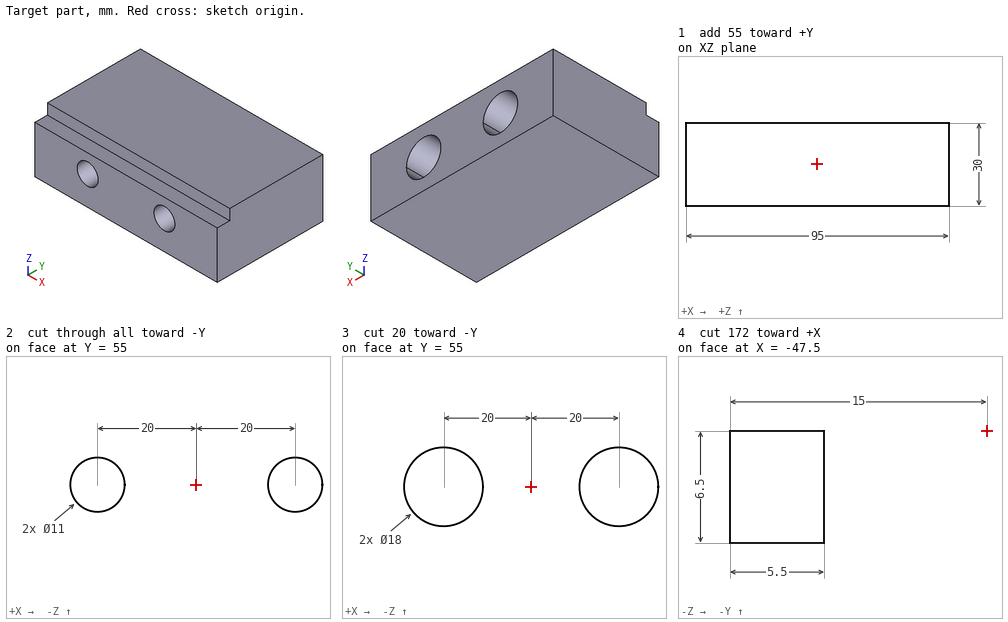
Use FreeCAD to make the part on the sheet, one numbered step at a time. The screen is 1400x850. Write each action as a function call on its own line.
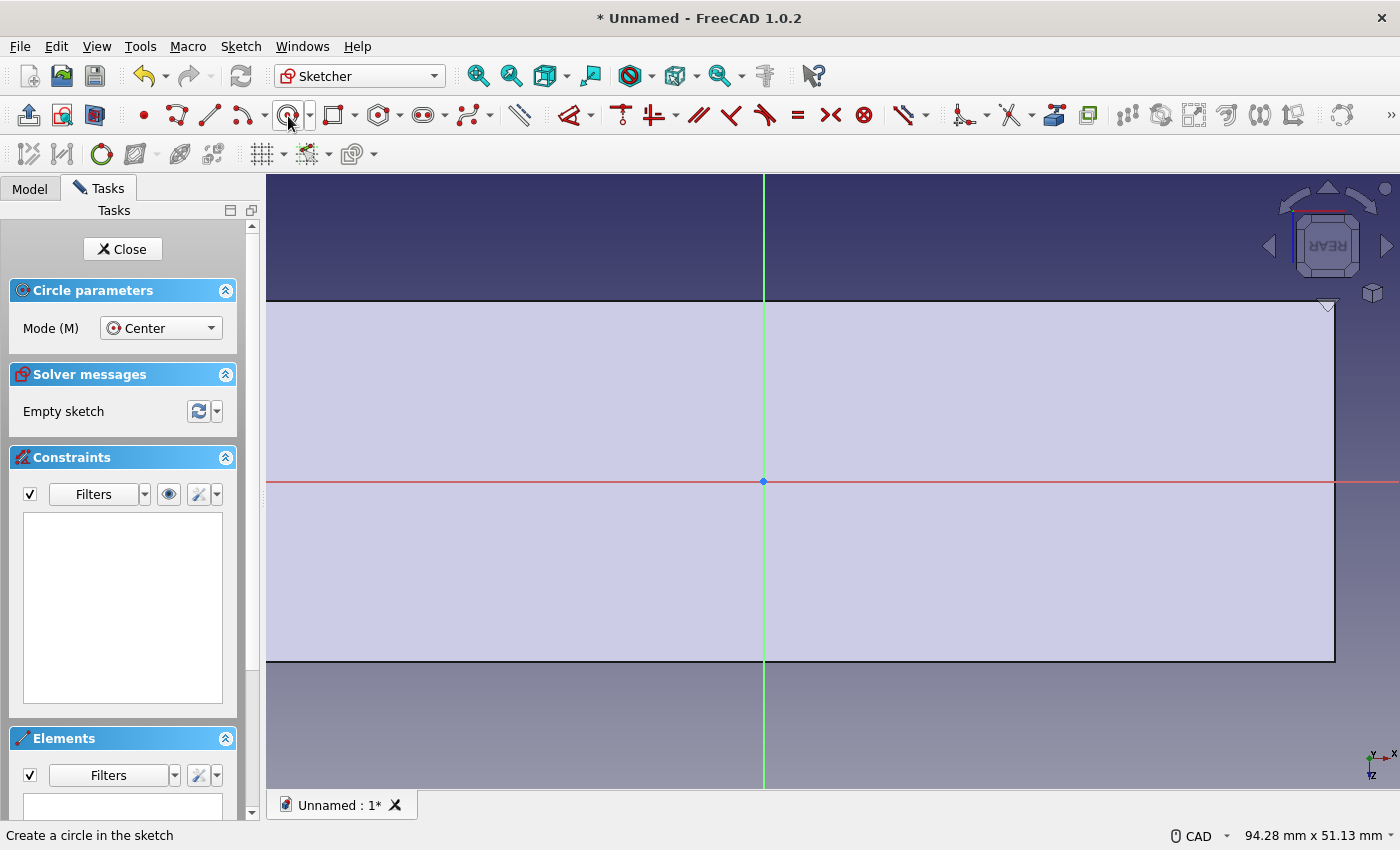
click(523, 481)
move(570, 435)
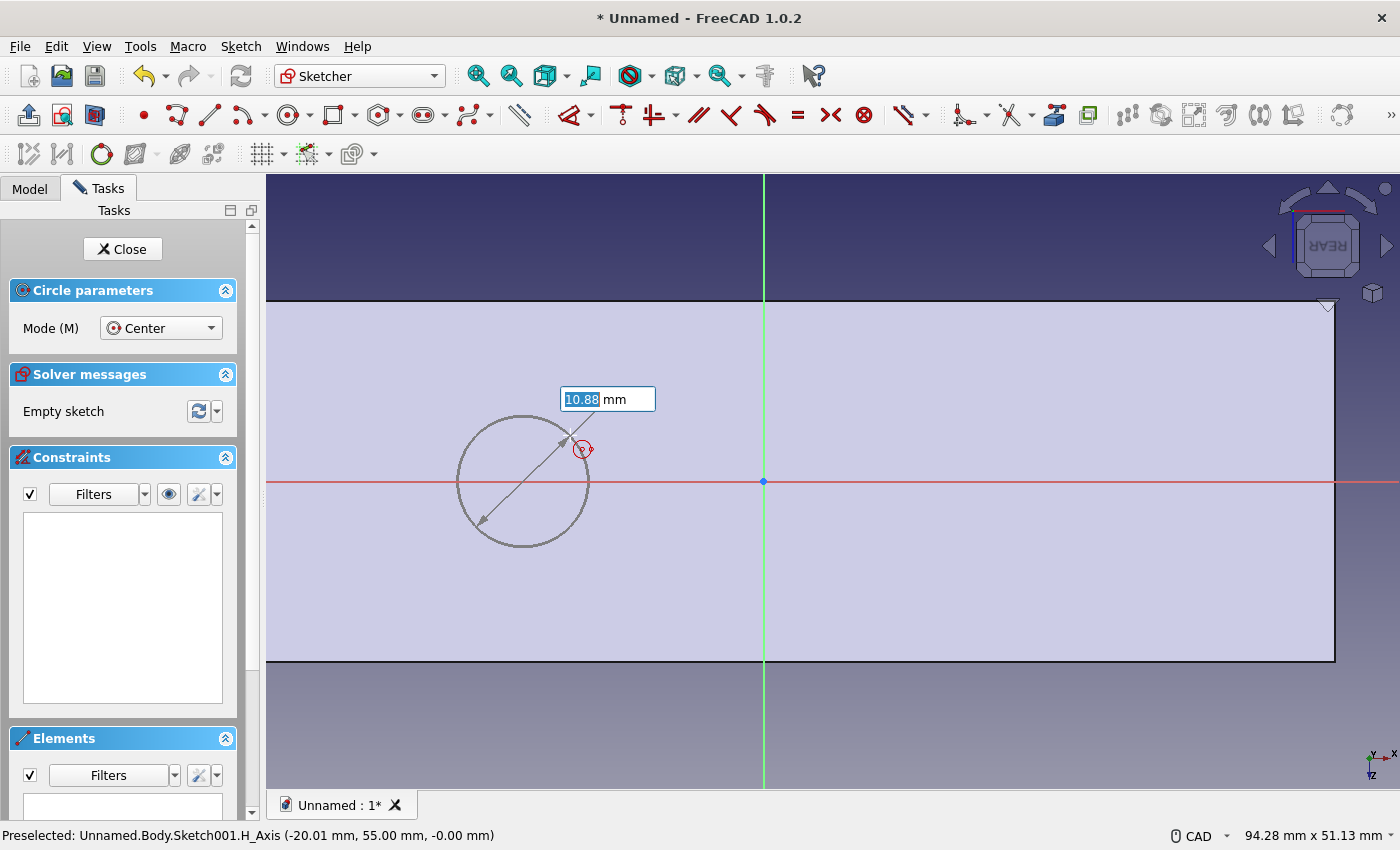
text(11)
key(Return)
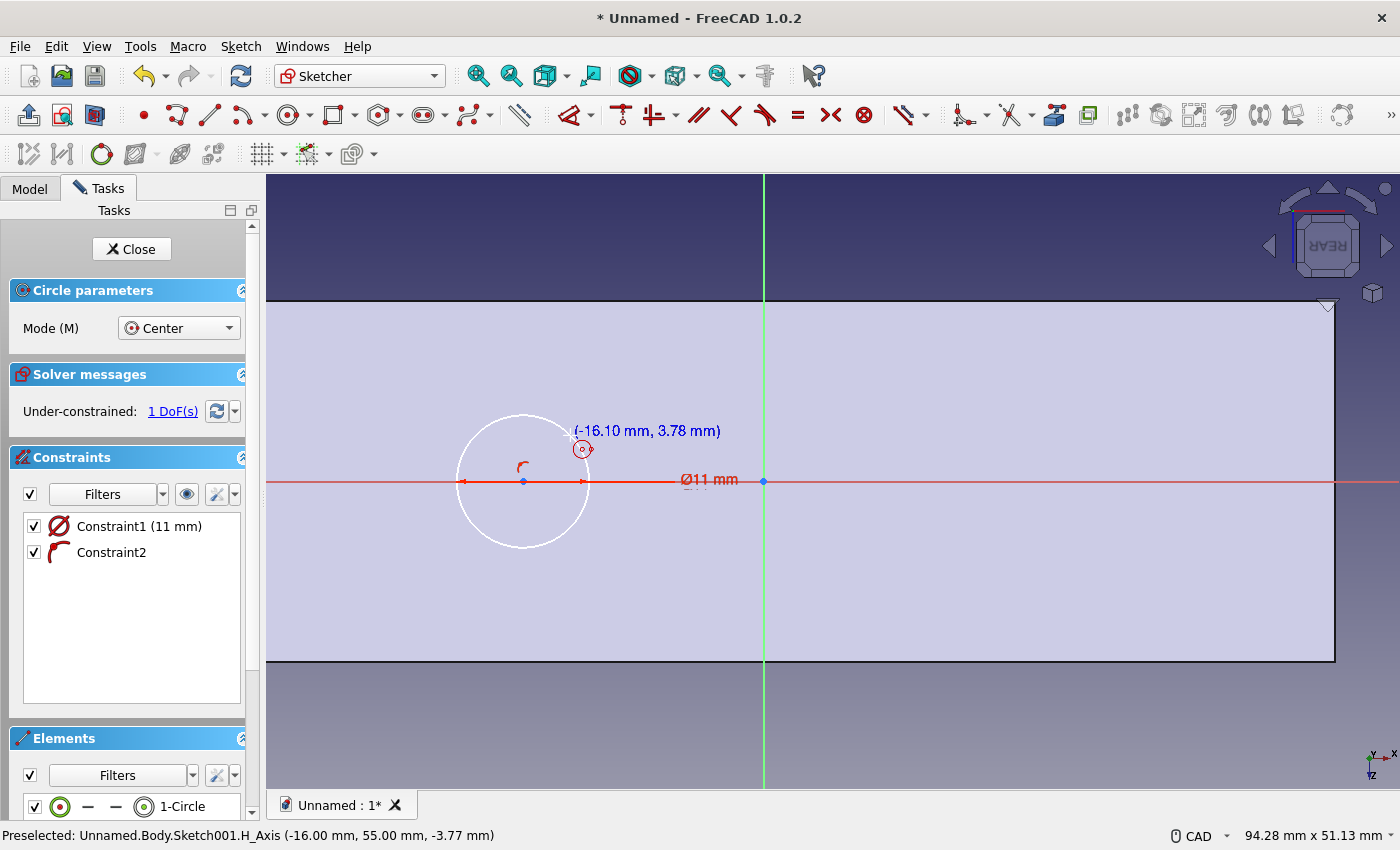
click(1004, 481)
move(1051, 435)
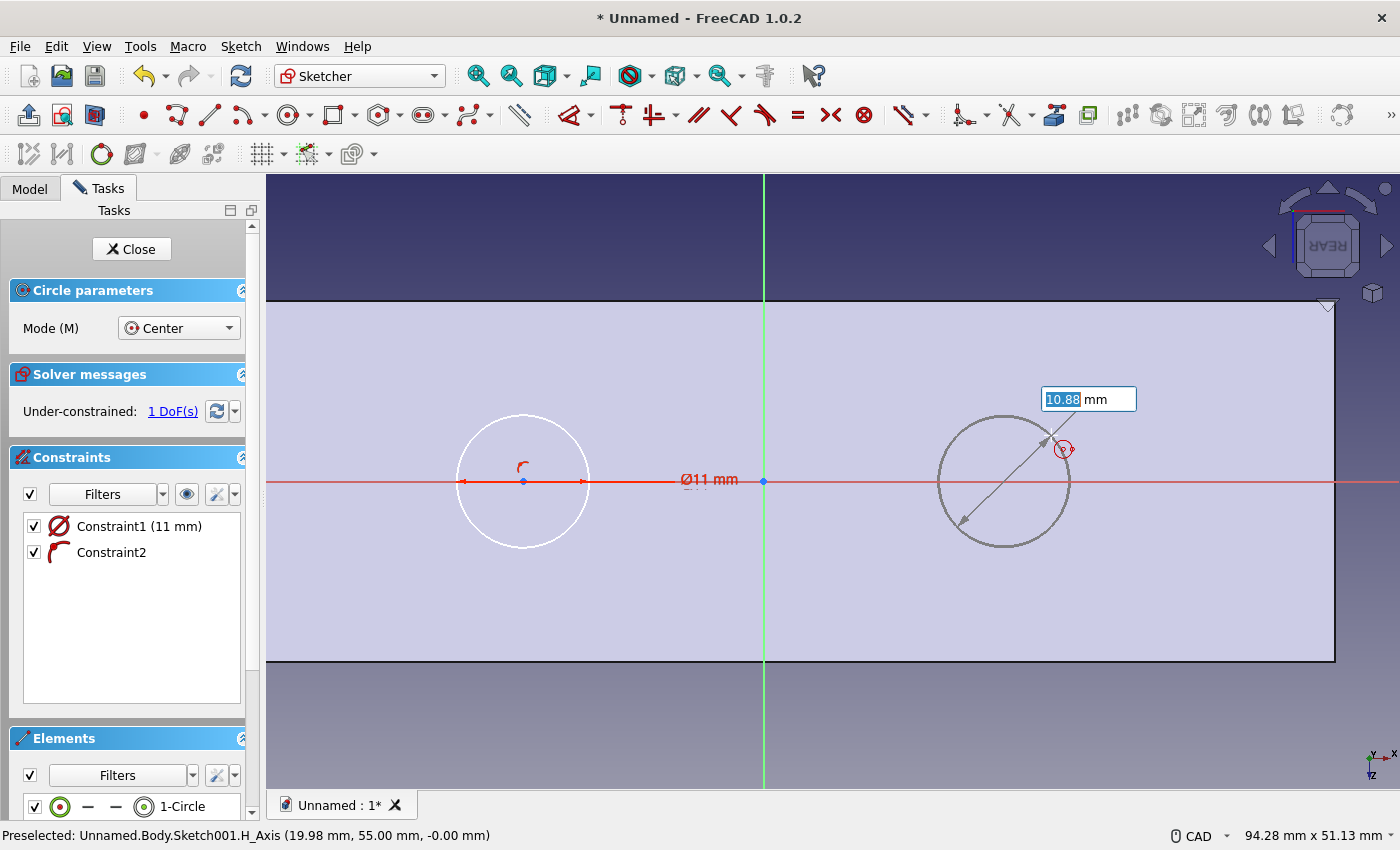
text(11)
key(Return)
key(Escape)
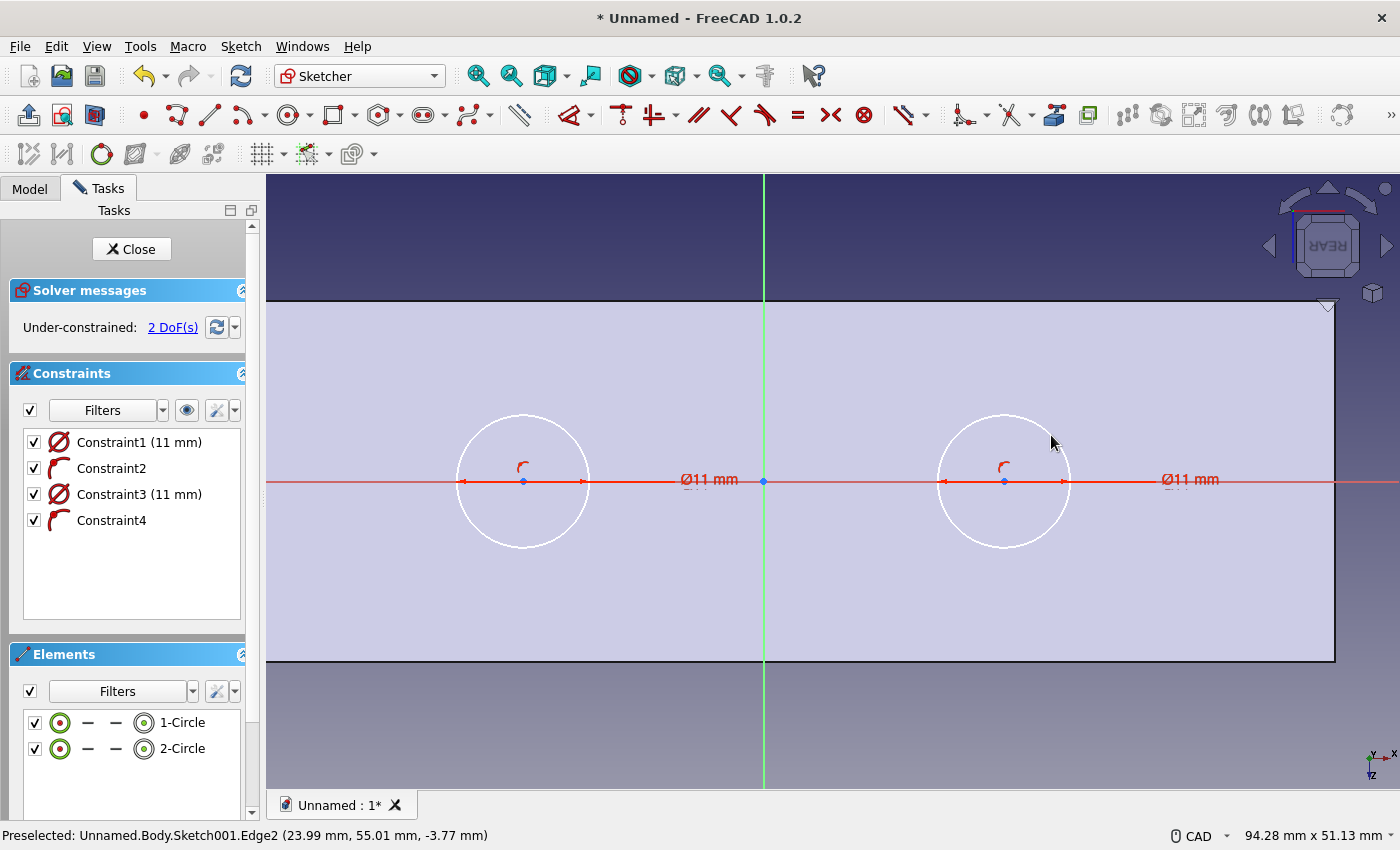
click(568, 116)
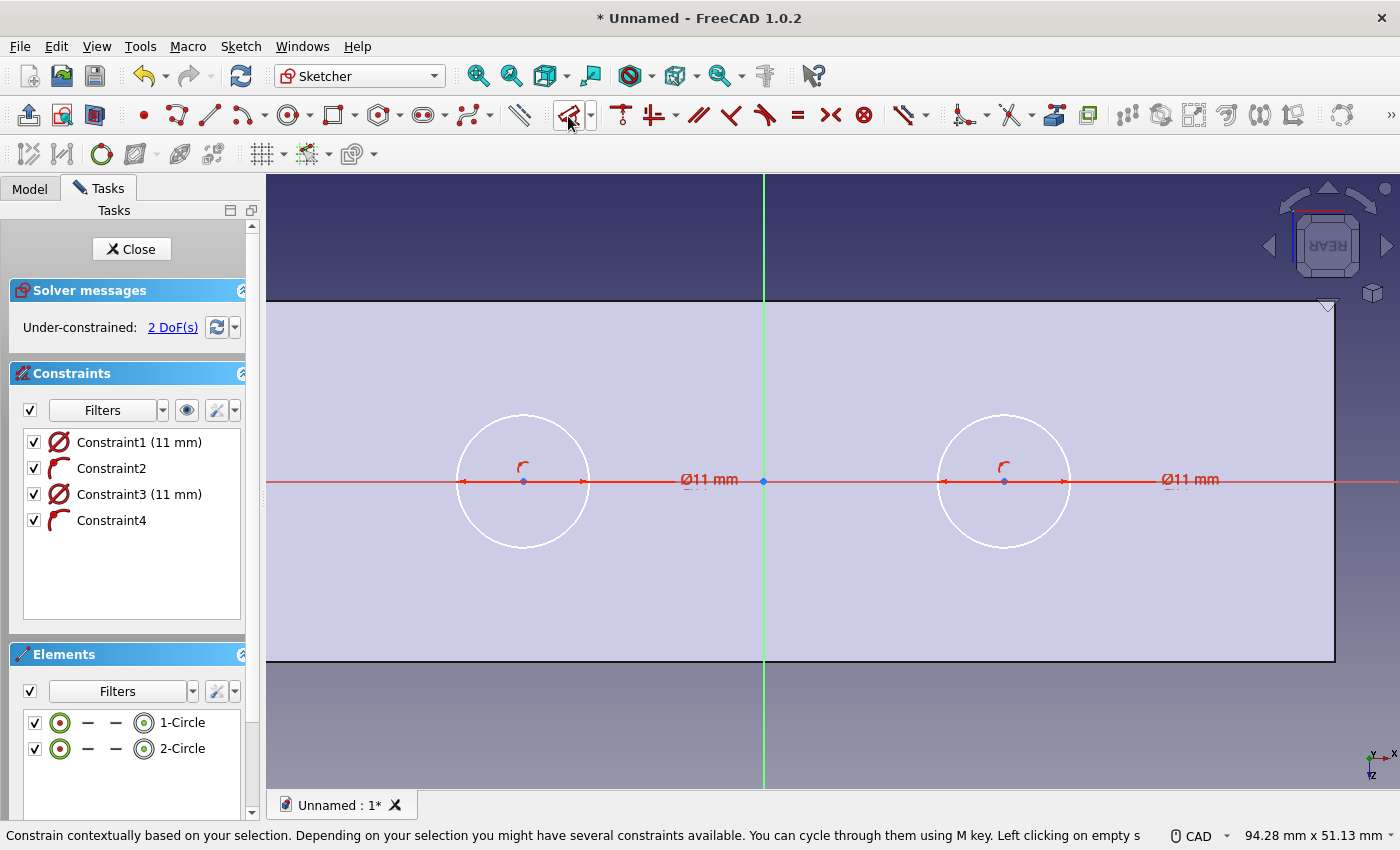
click(523, 481)
click(643, 515)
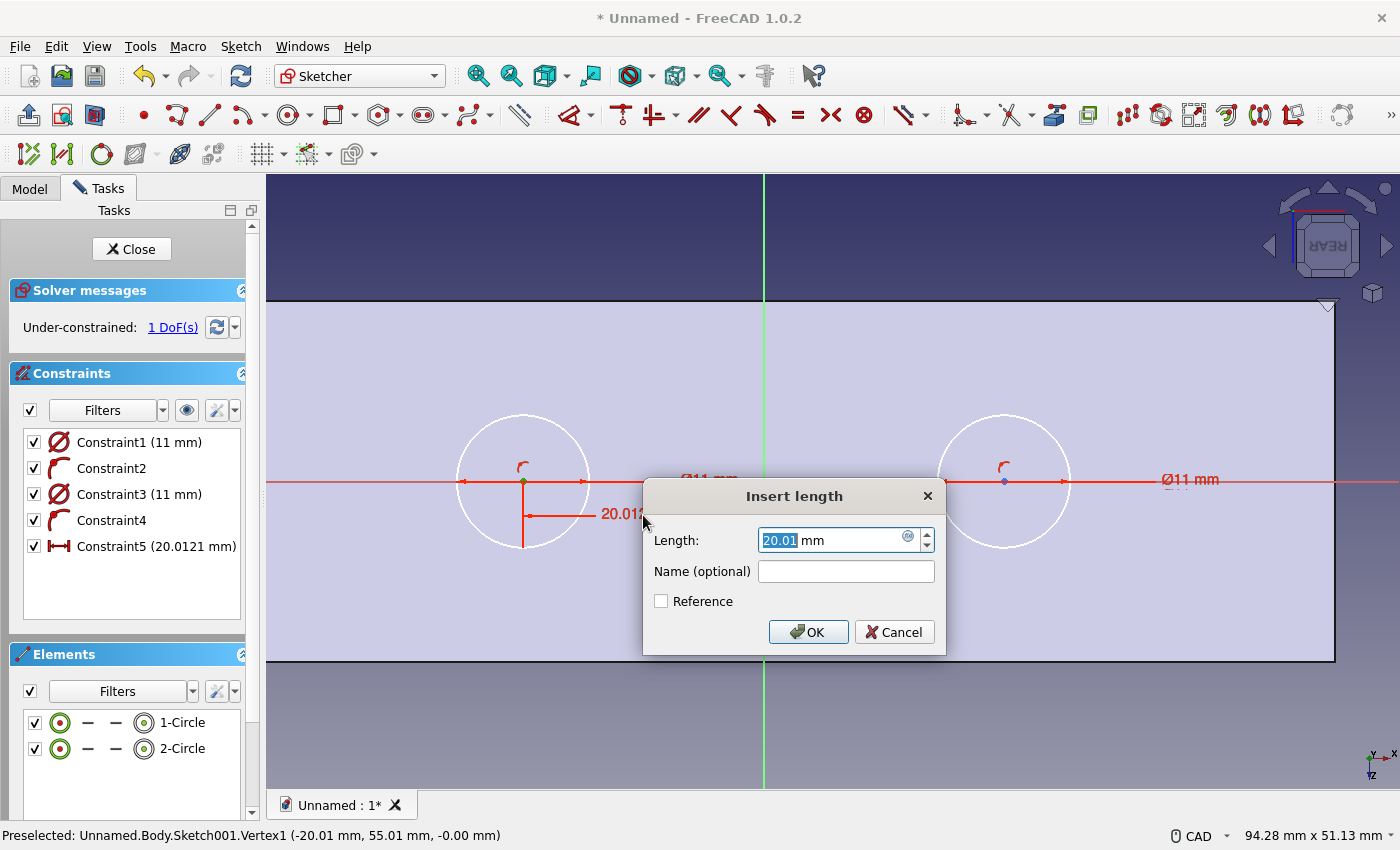
text(20)
key(Return)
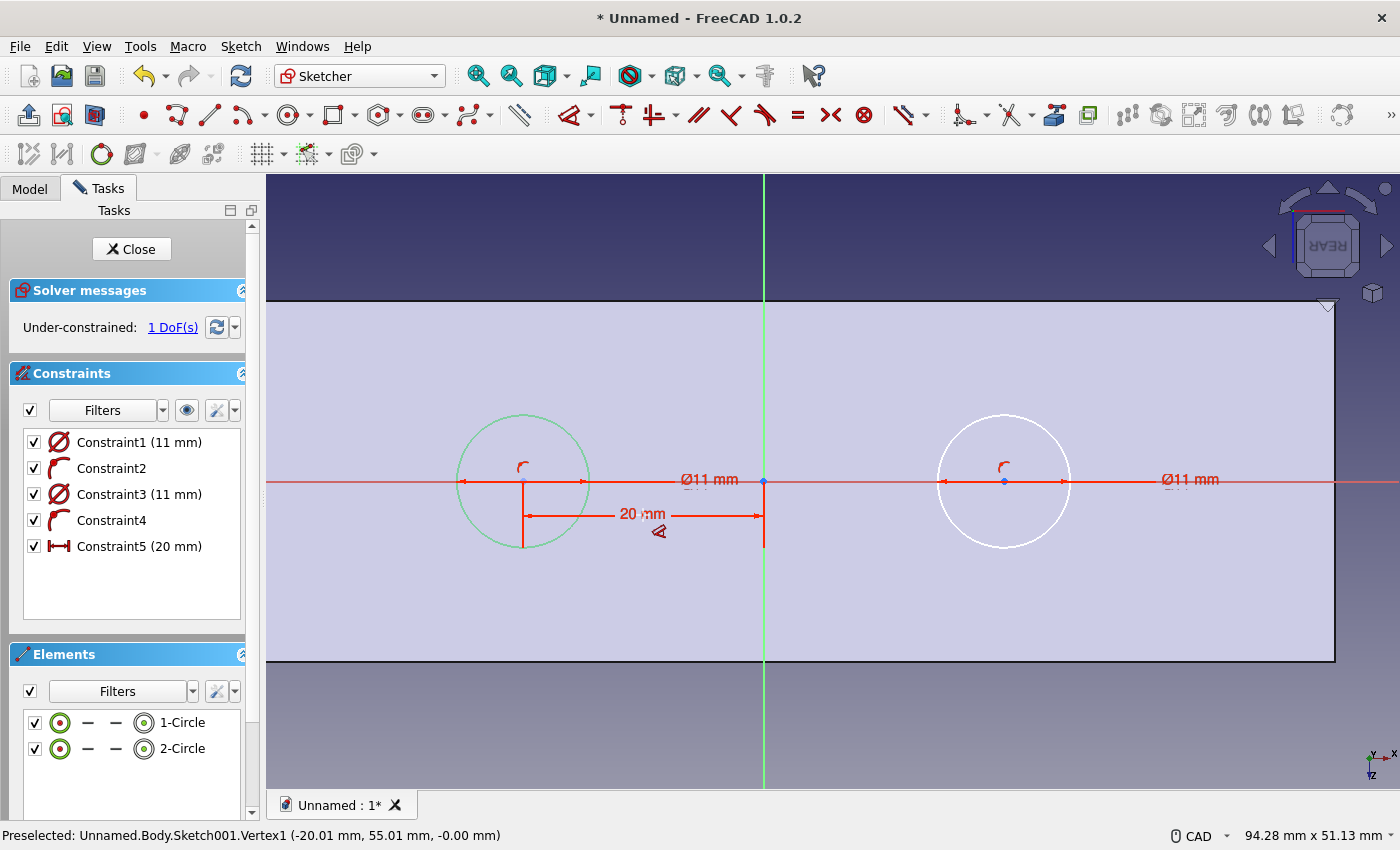
click(1004, 481)
click(884, 515)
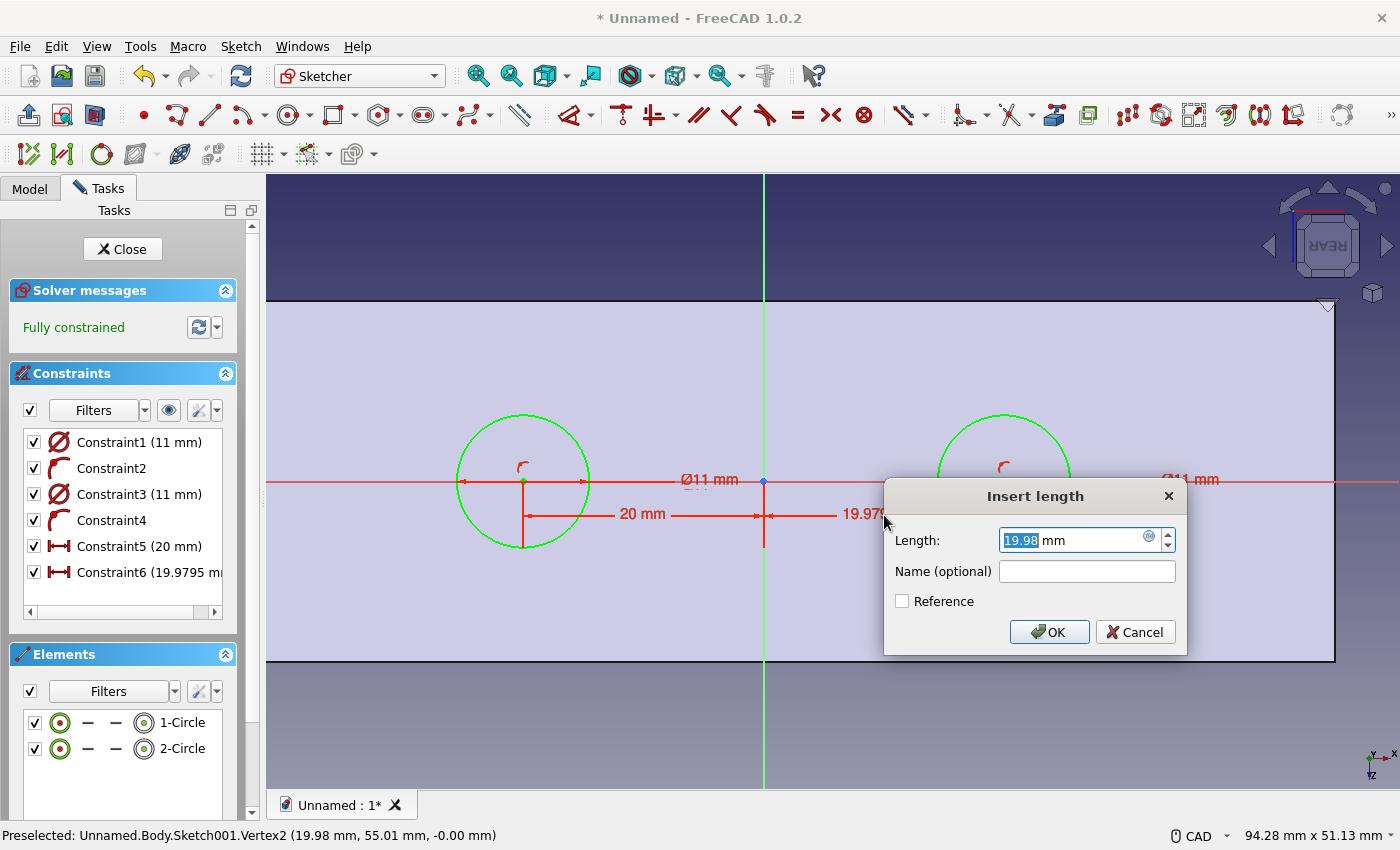
text(20)
key(Return)
key(Escape)